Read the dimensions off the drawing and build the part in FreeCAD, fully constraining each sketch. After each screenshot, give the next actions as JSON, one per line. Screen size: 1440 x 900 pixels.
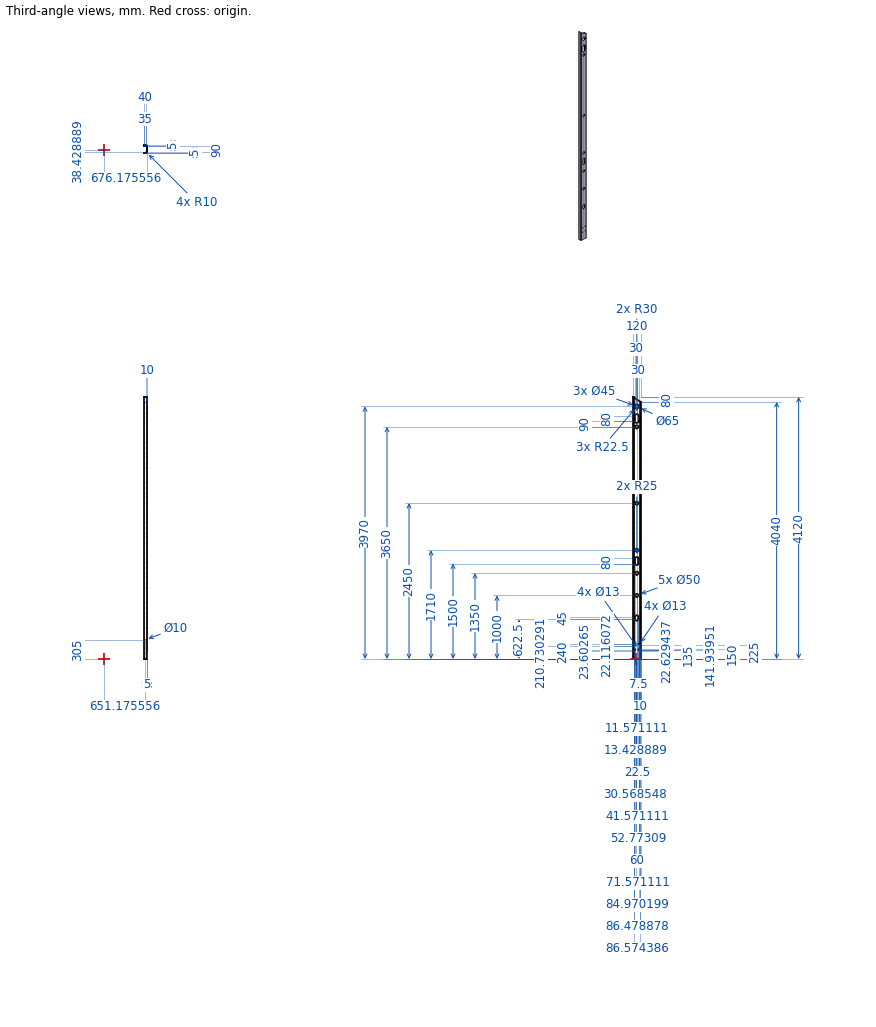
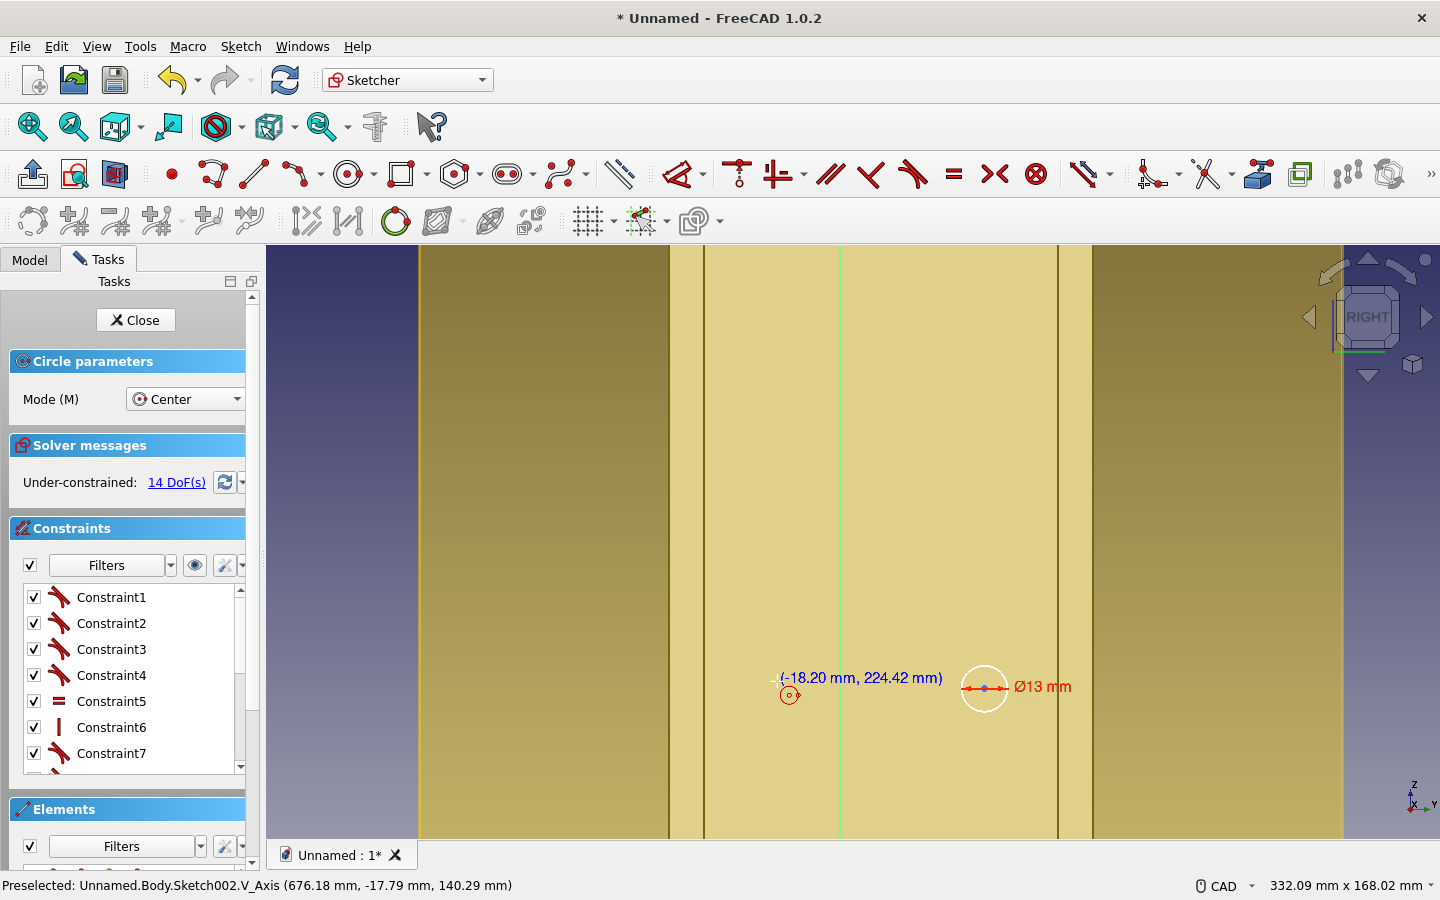
{"action": "scroll", "coordinate": [781, 753], "scroll_direction": "down", "scroll_amount": 17}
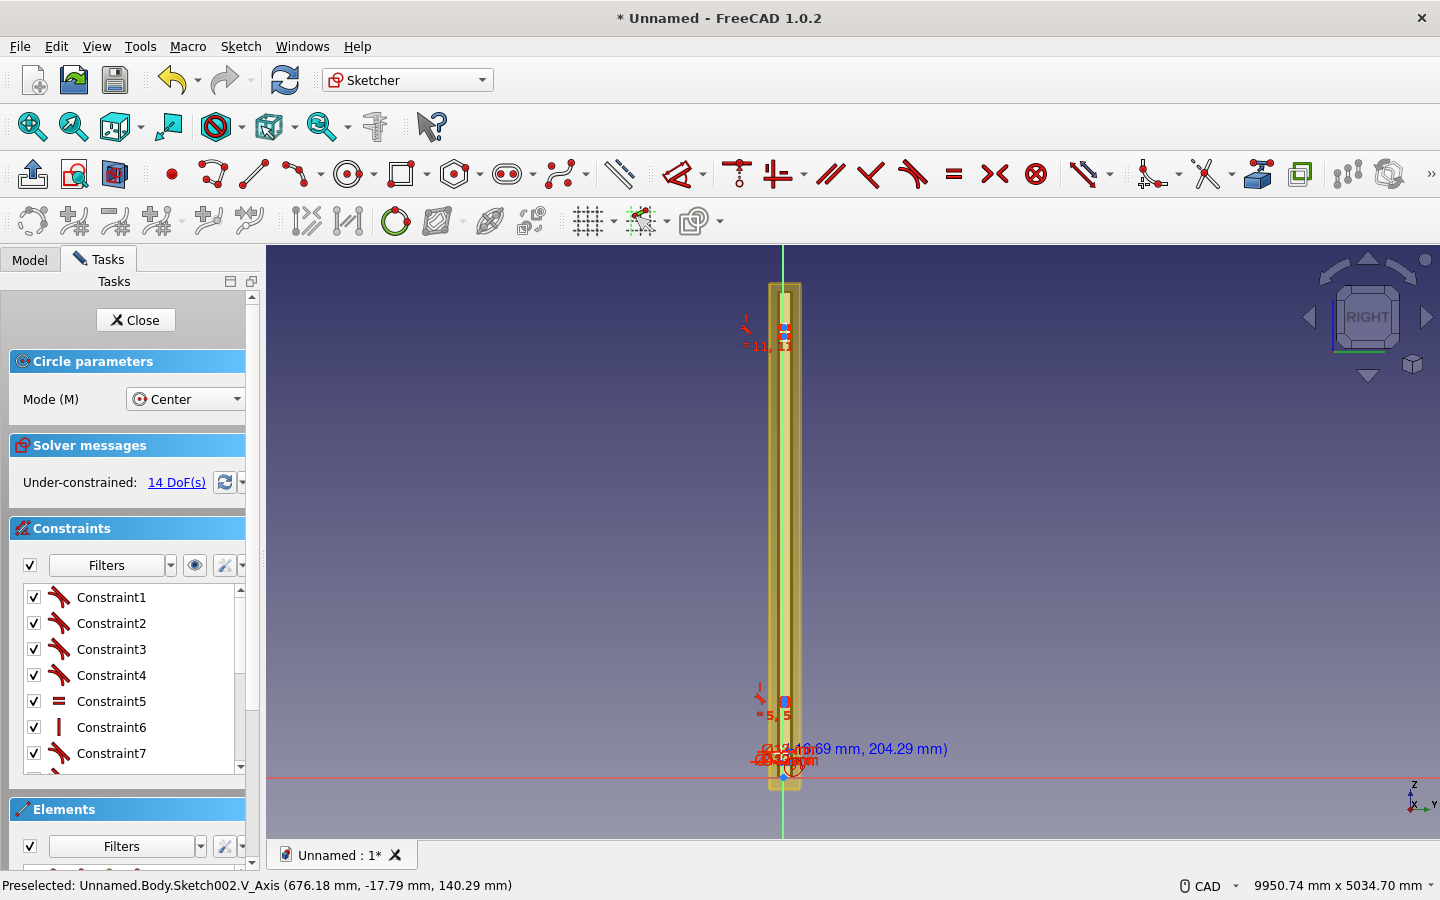
{"action": "scroll", "coordinate": [781, 751], "scroll_direction": "up", "scroll_amount": 10}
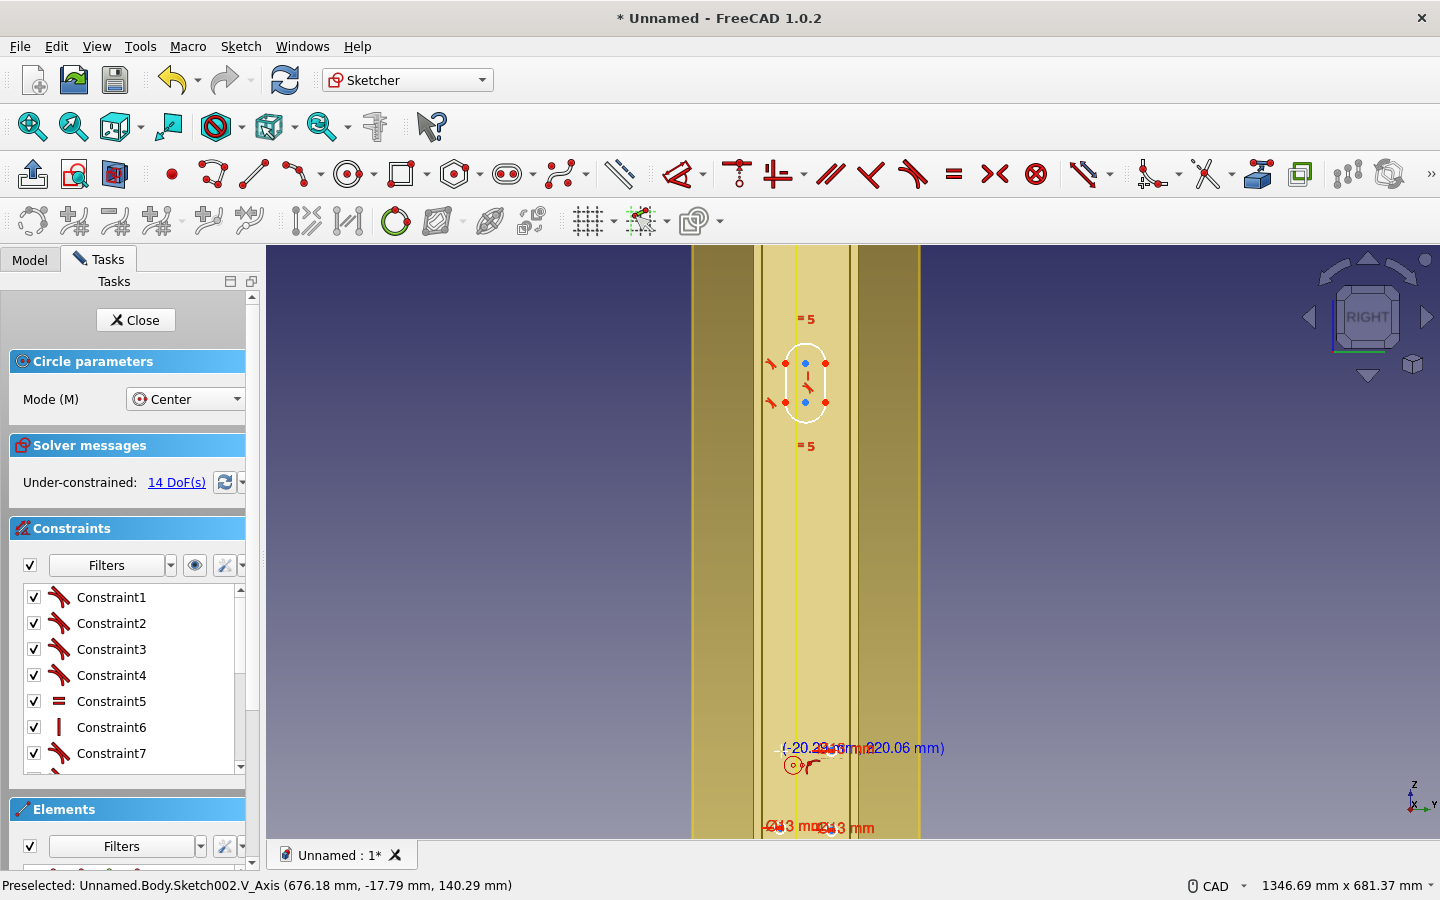
{"action": "left_click", "coordinate": [780, 749]}
{"action": "mouse_move", "coordinate": [776, 745]}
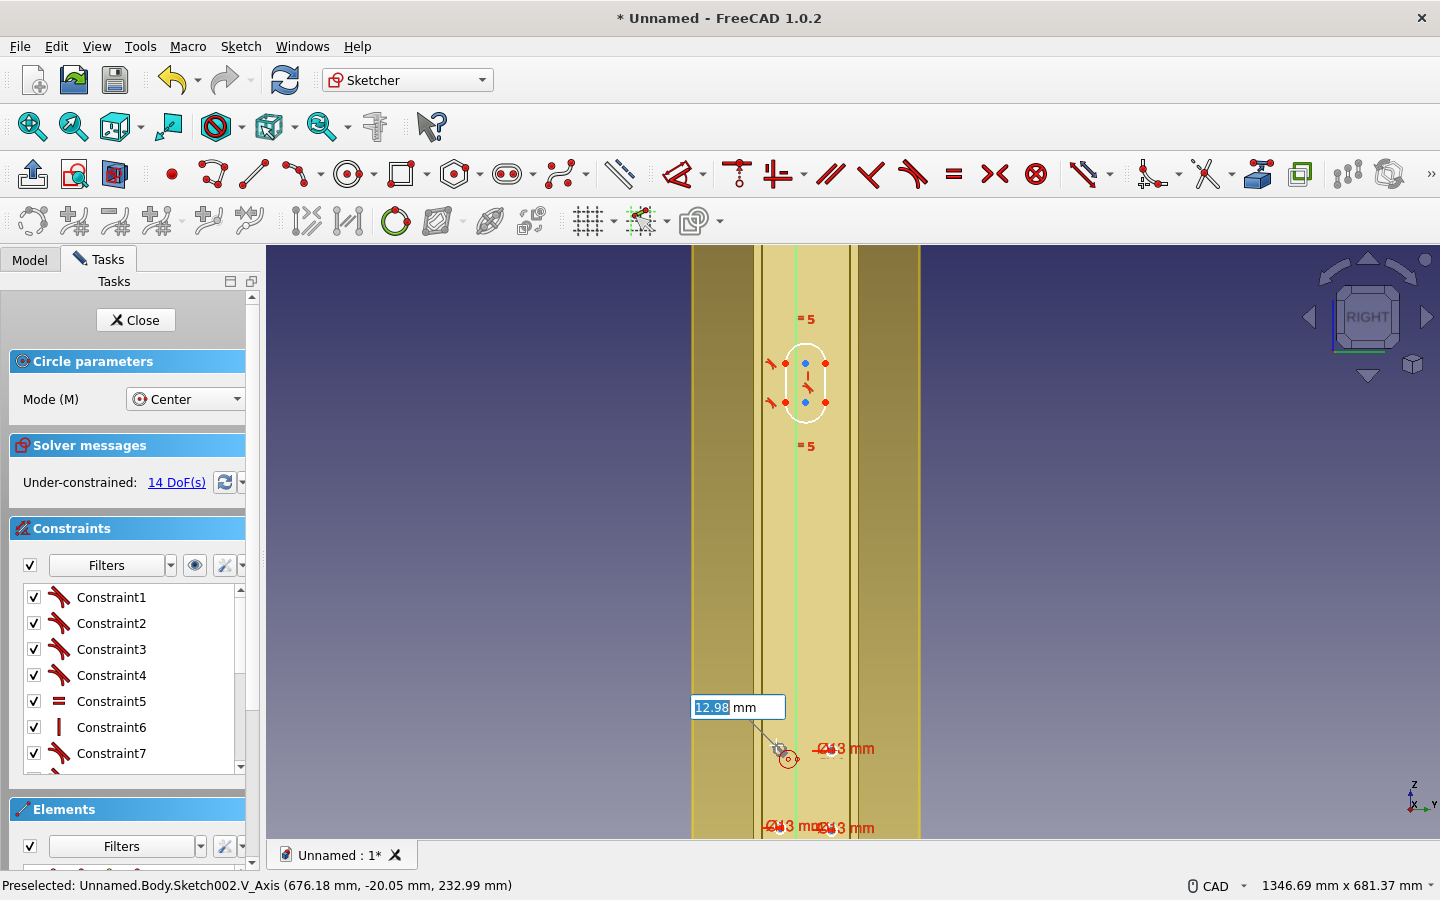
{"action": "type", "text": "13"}
{"action": "key", "text": "Return"}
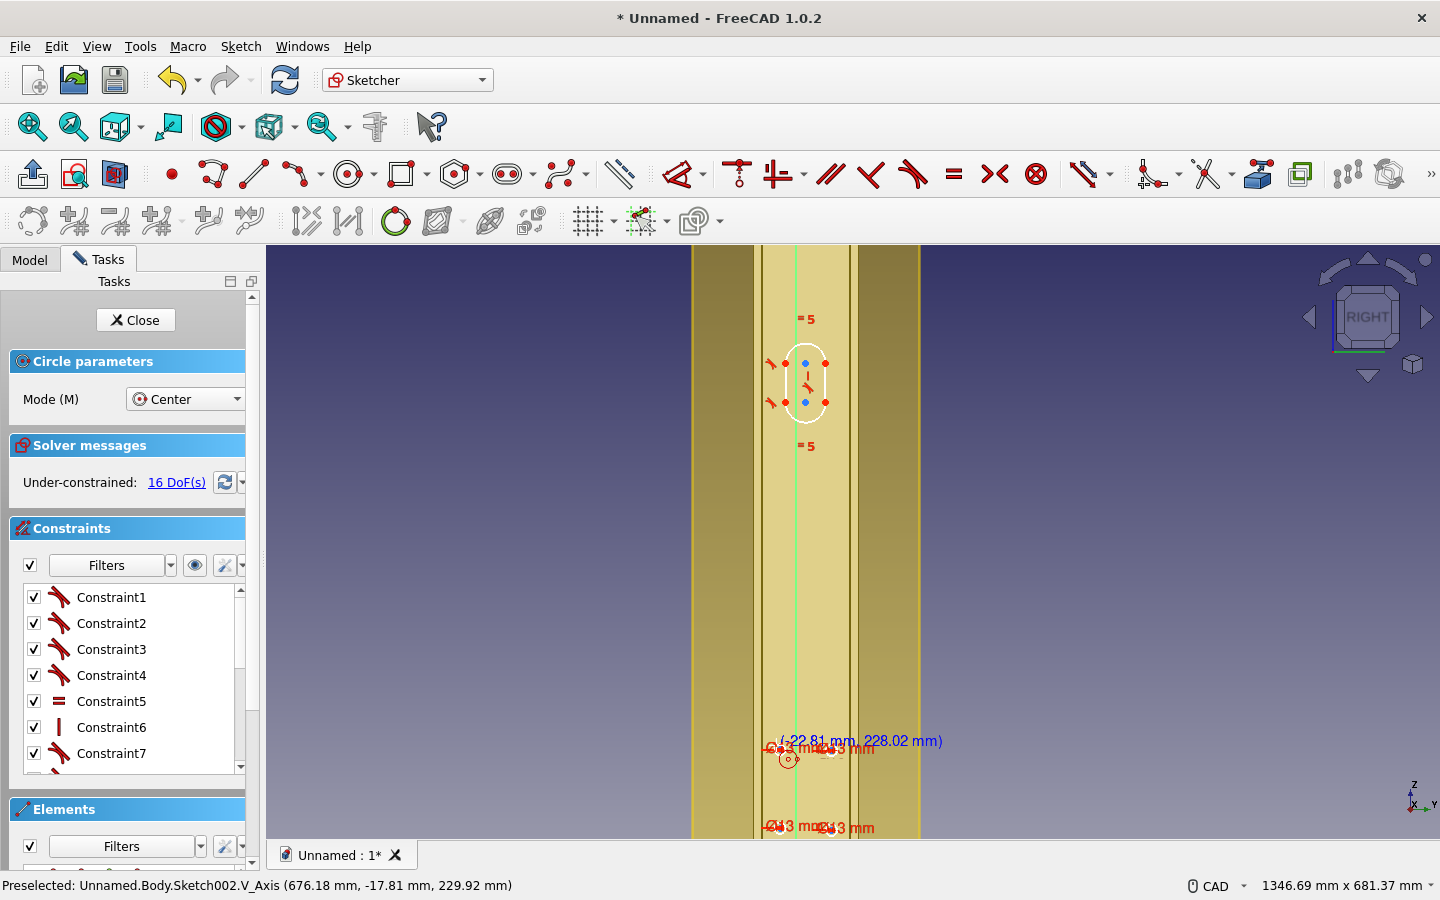
{"action": "scroll", "coordinate": [782, 709], "scroll_direction": "down", "scroll_amount": 11}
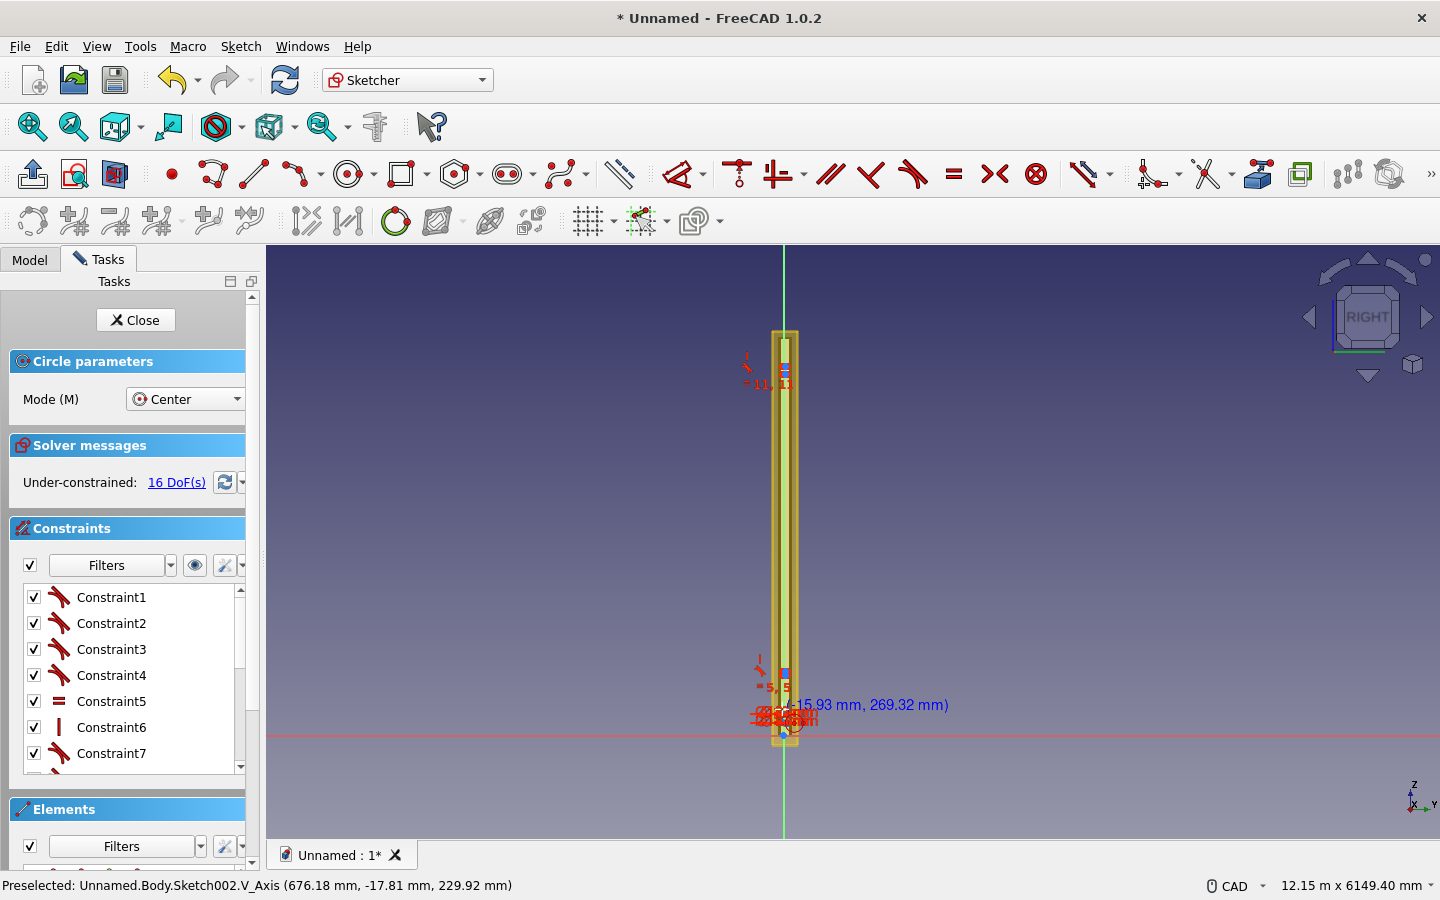
{"action": "scroll", "coordinate": [785, 639], "scroll_direction": "up", "scroll_amount": 14}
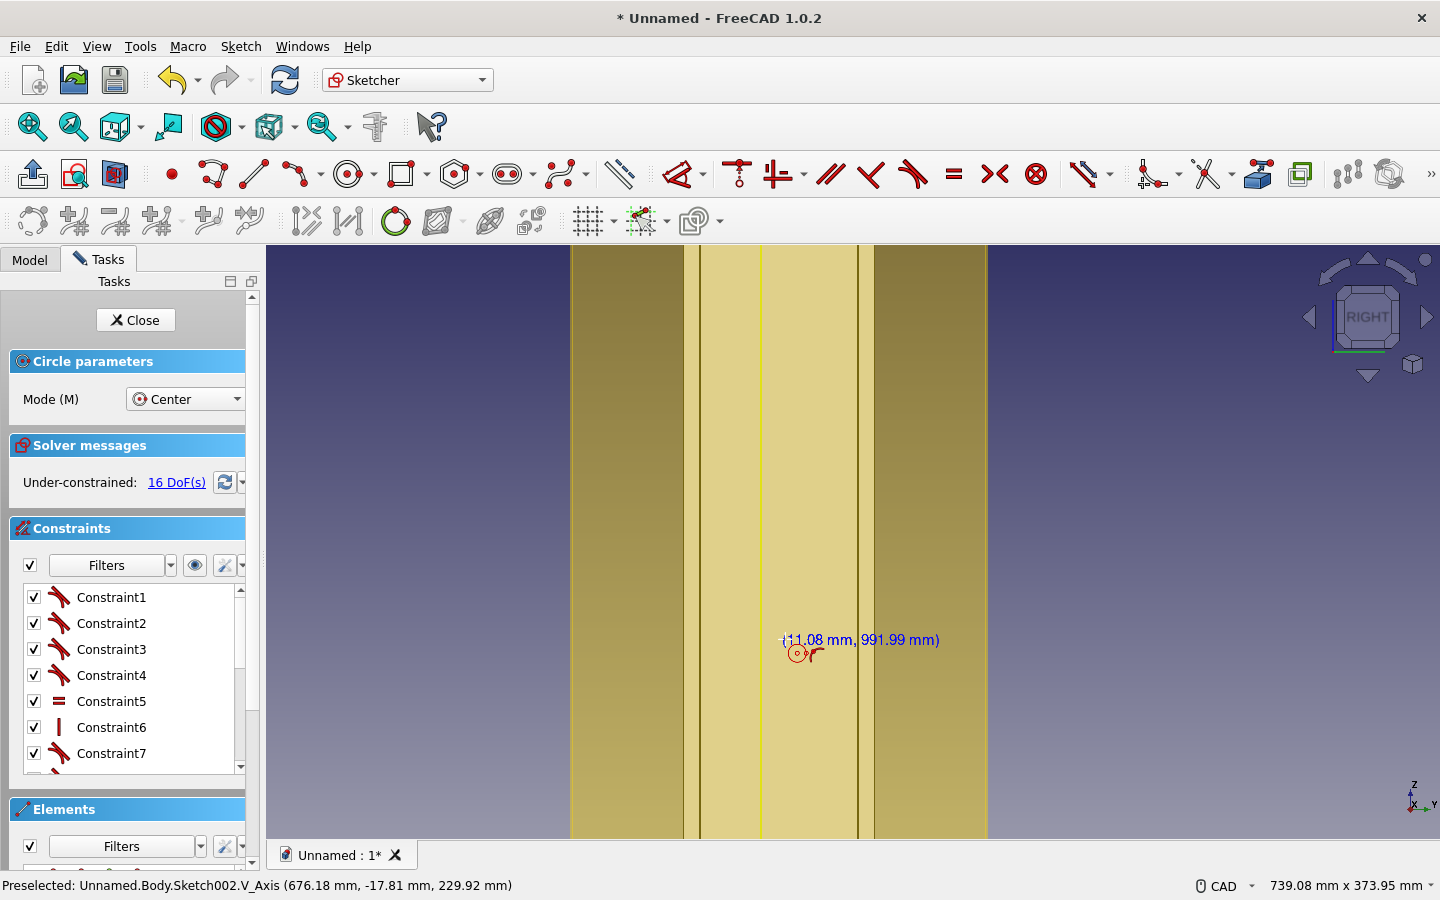
{"action": "left_click", "coordinate": [779, 632]}